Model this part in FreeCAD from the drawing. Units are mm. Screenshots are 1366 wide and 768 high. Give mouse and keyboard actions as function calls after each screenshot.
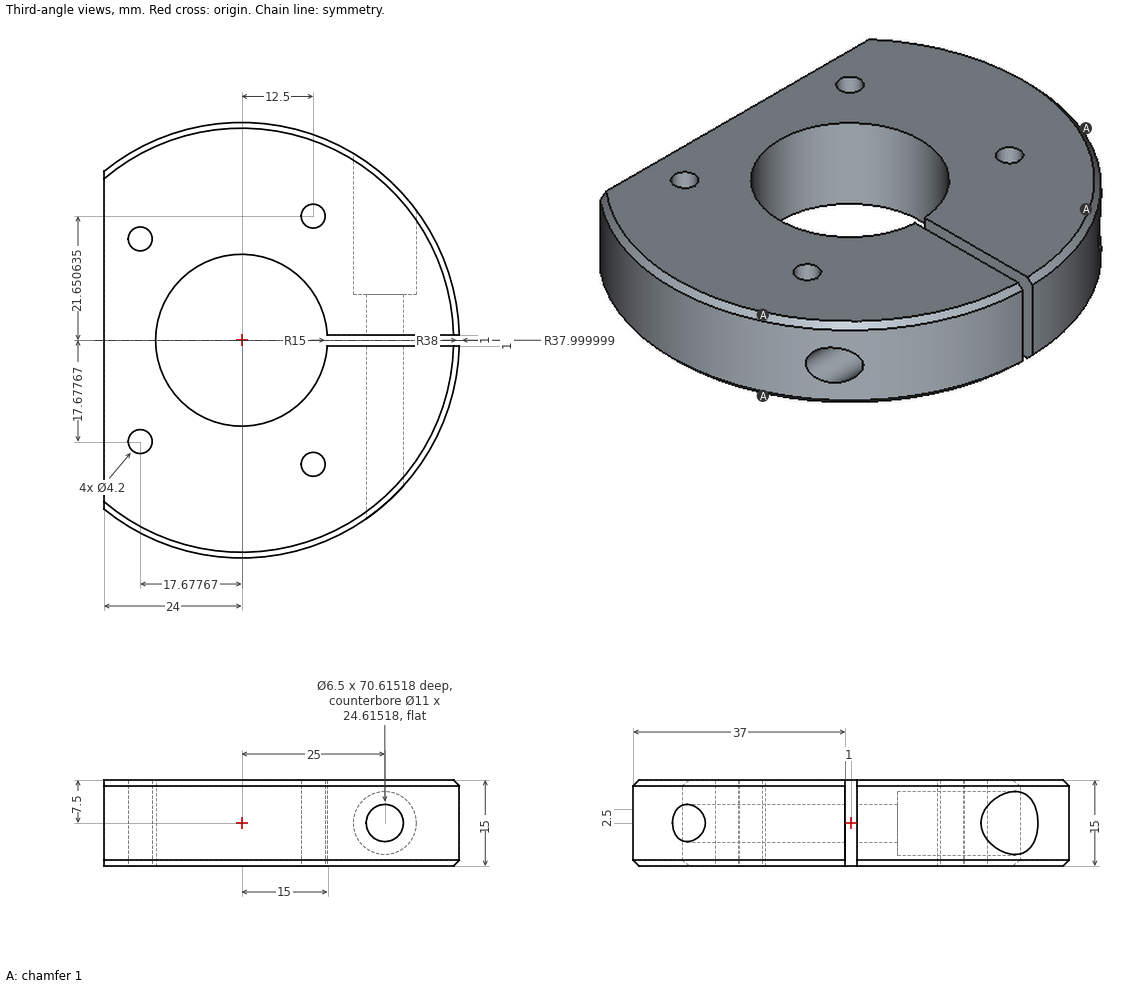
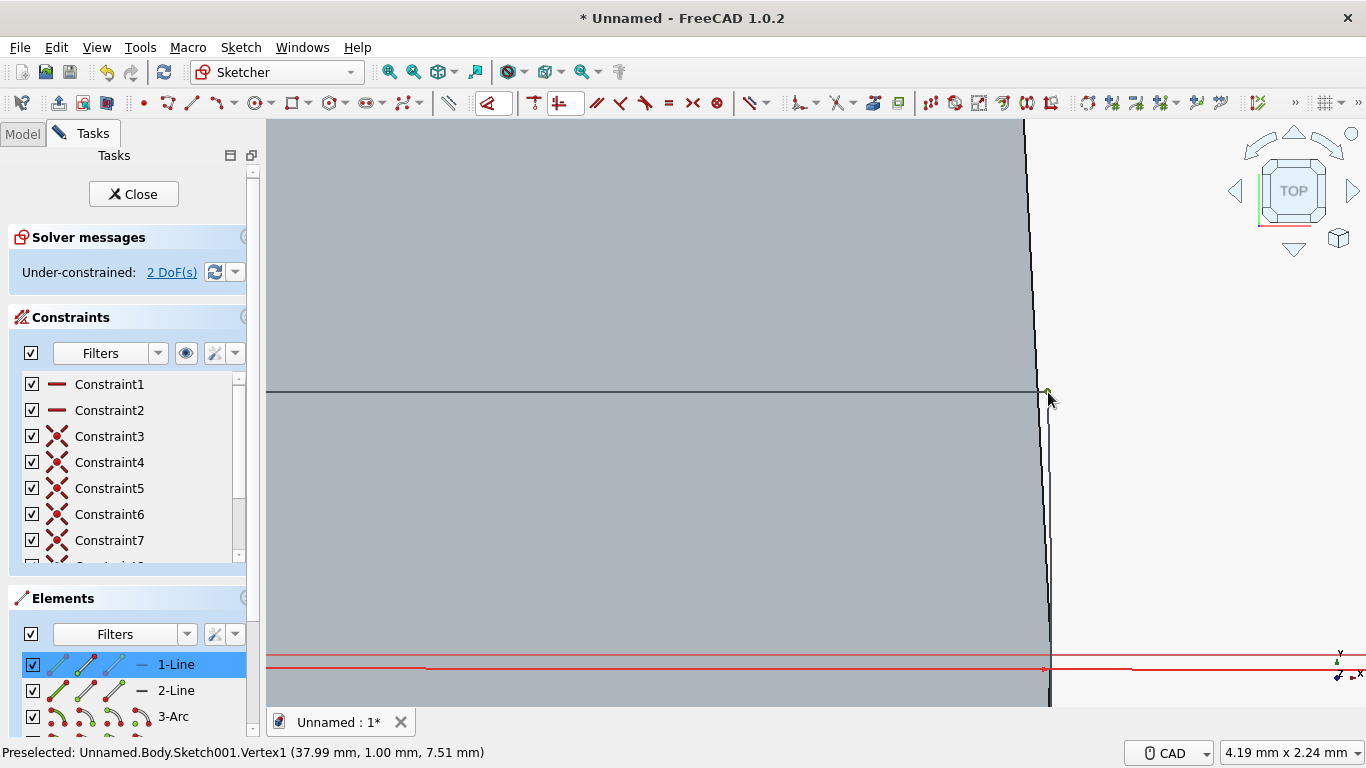
click(506, 104)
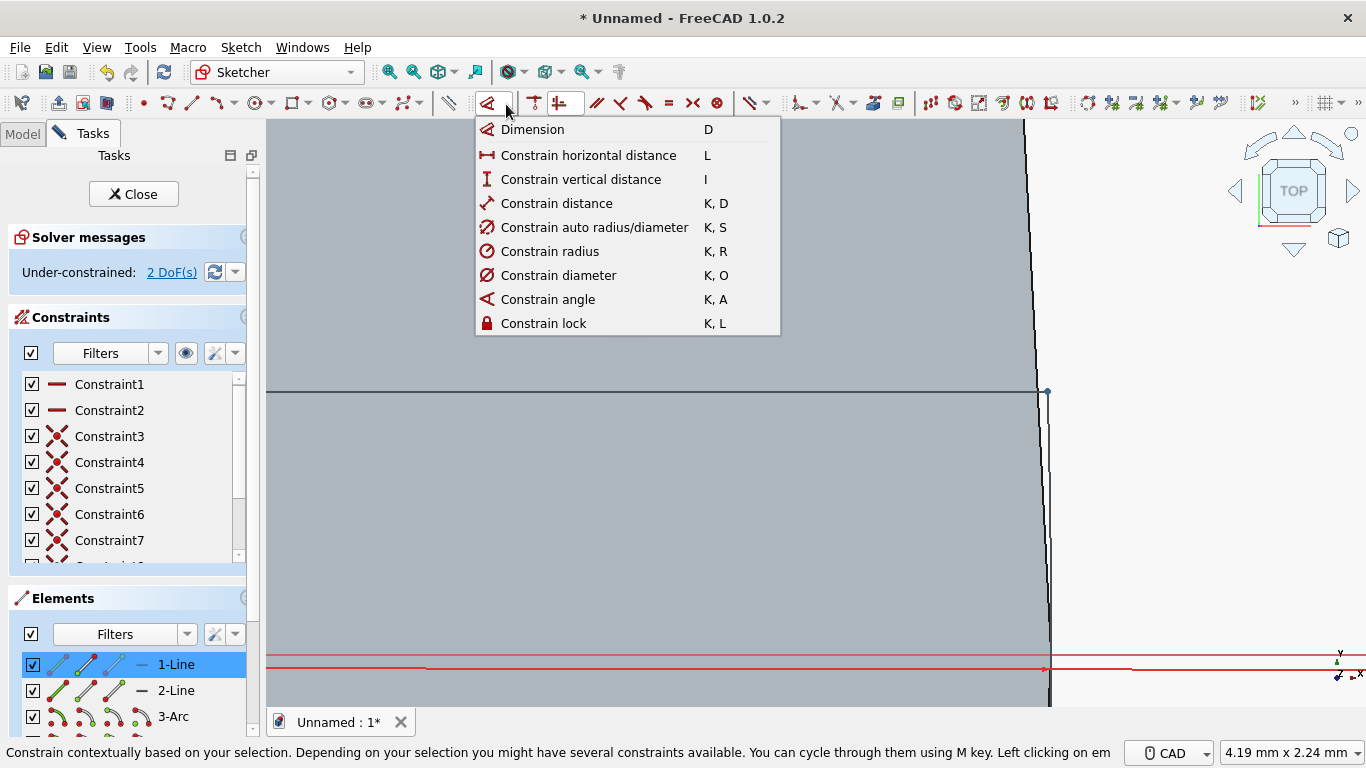
click(628, 179)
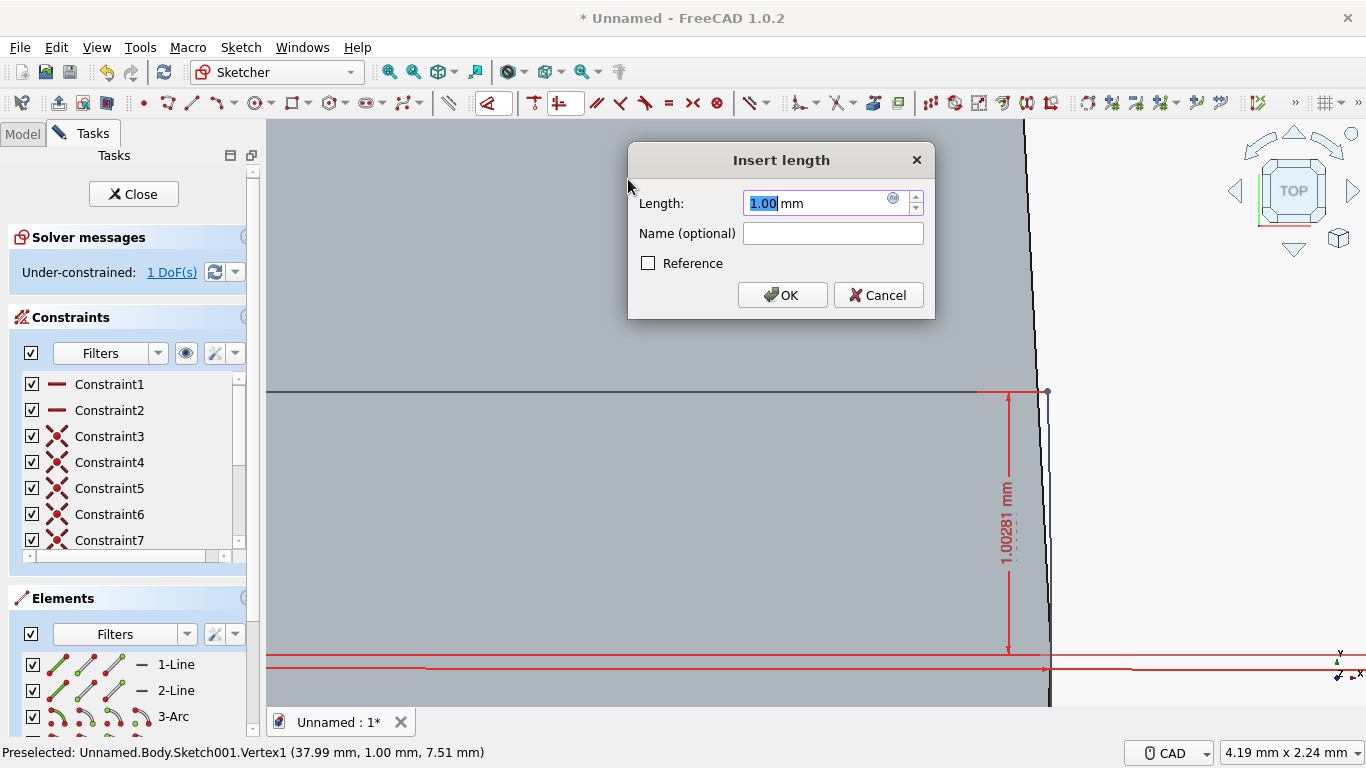
text(1)
key(Return)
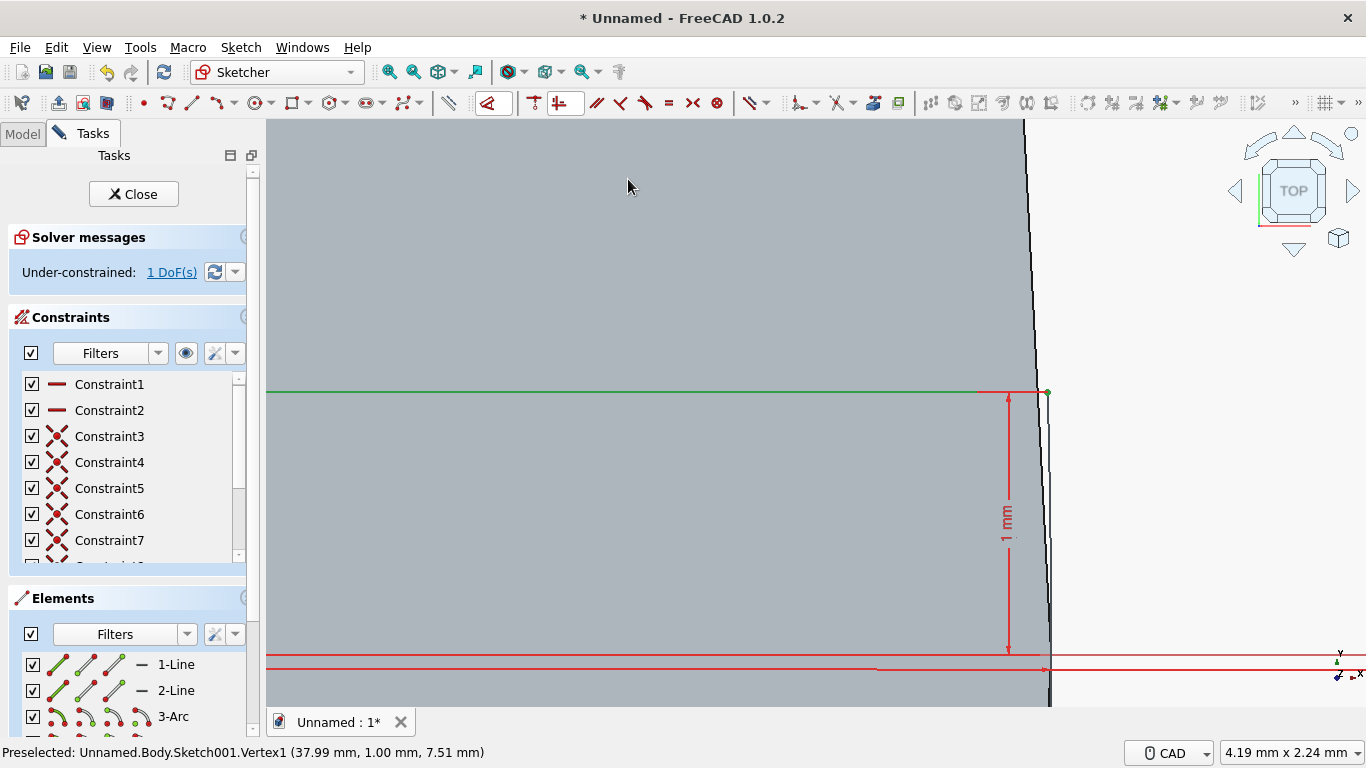
scroll(1051, 397, down, 14)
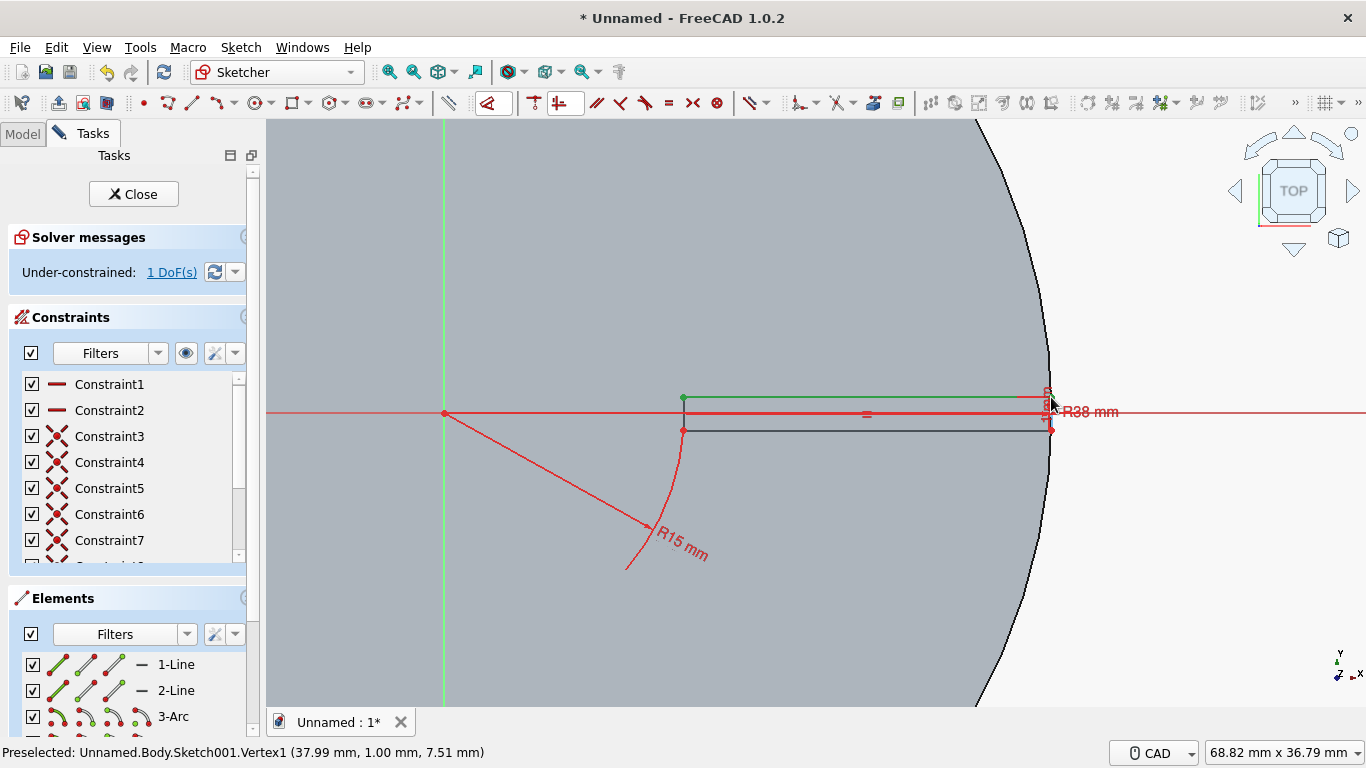
scroll(683, 431, up, 5)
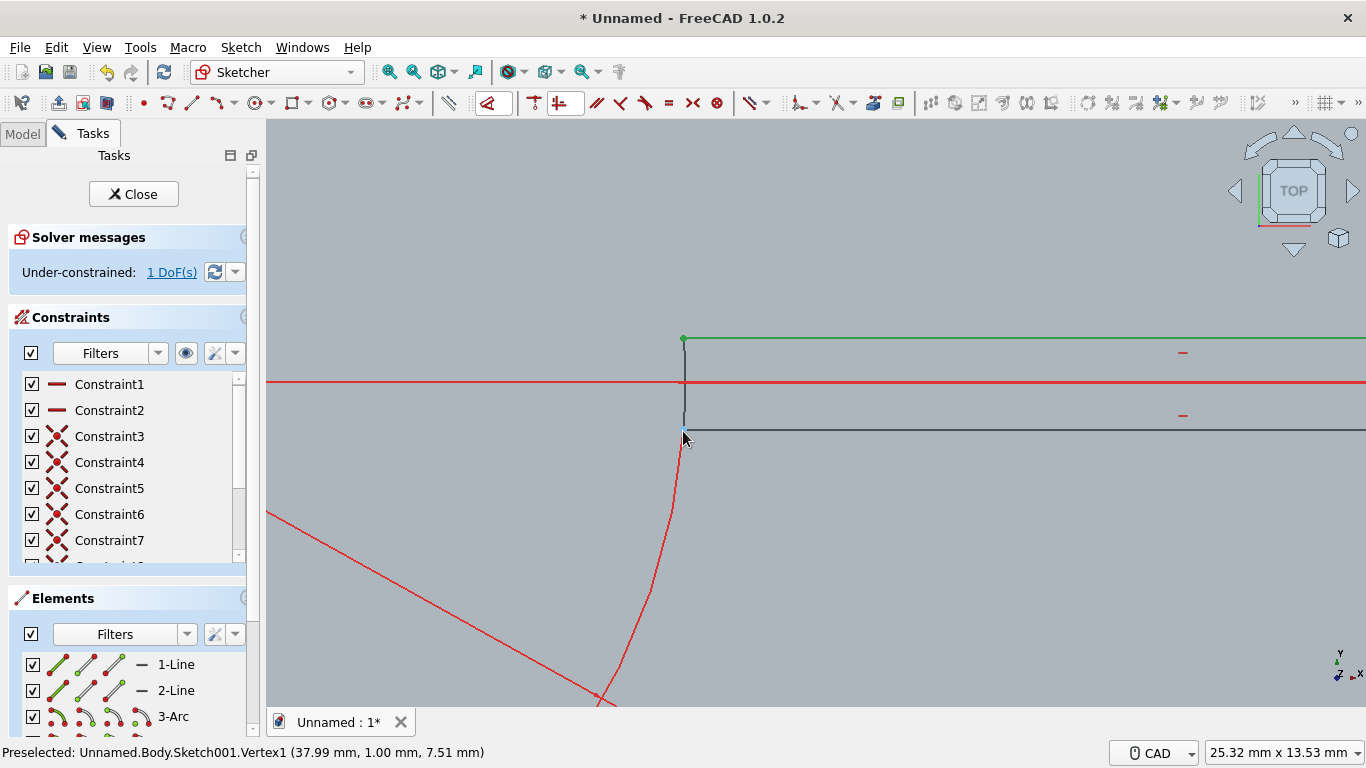
click(683, 430)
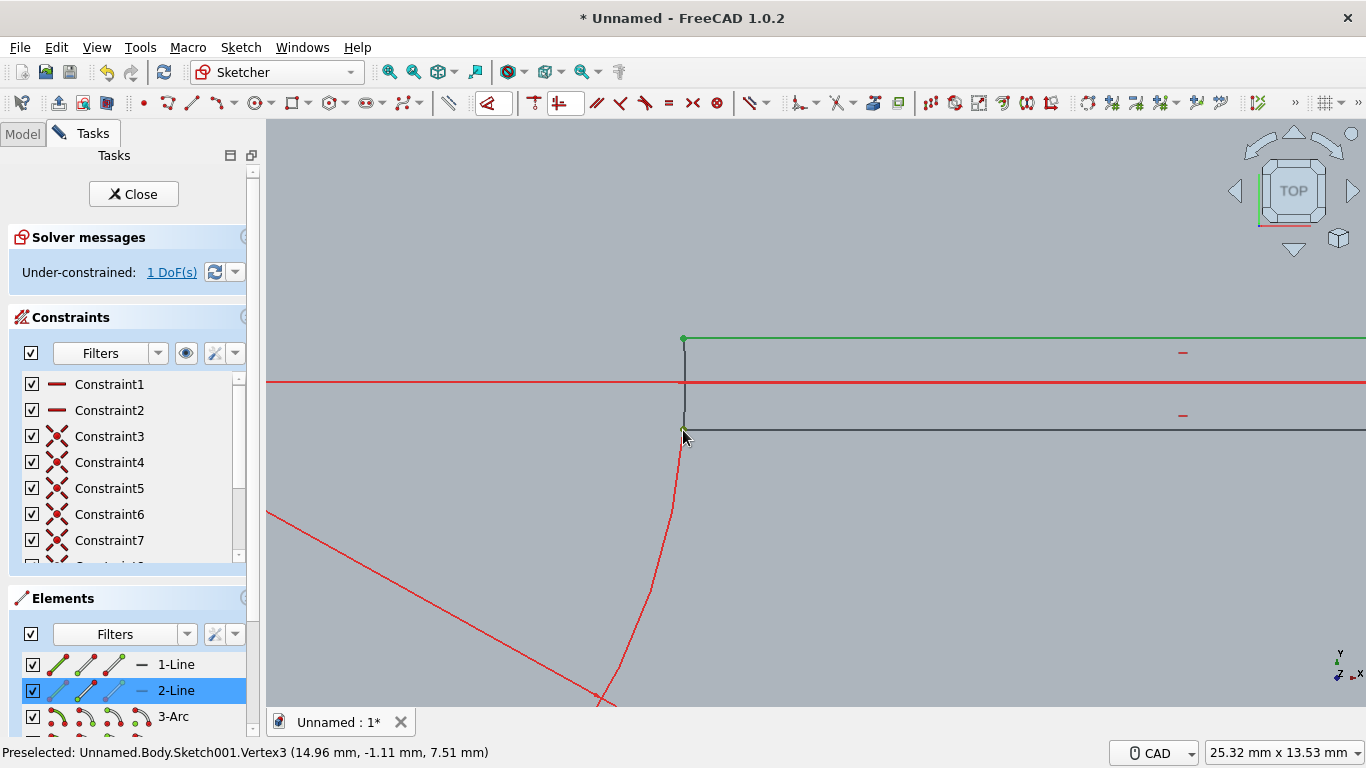
click(506, 104)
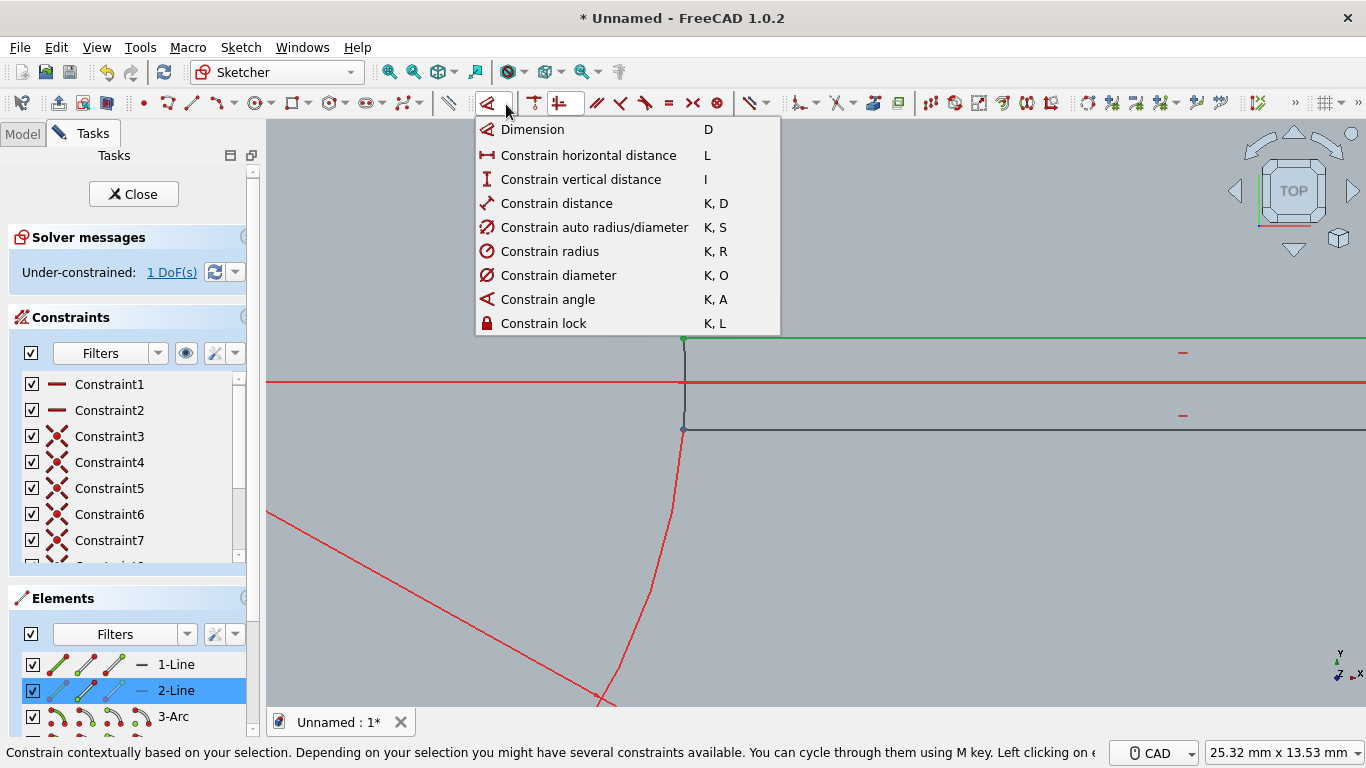
click(628, 179)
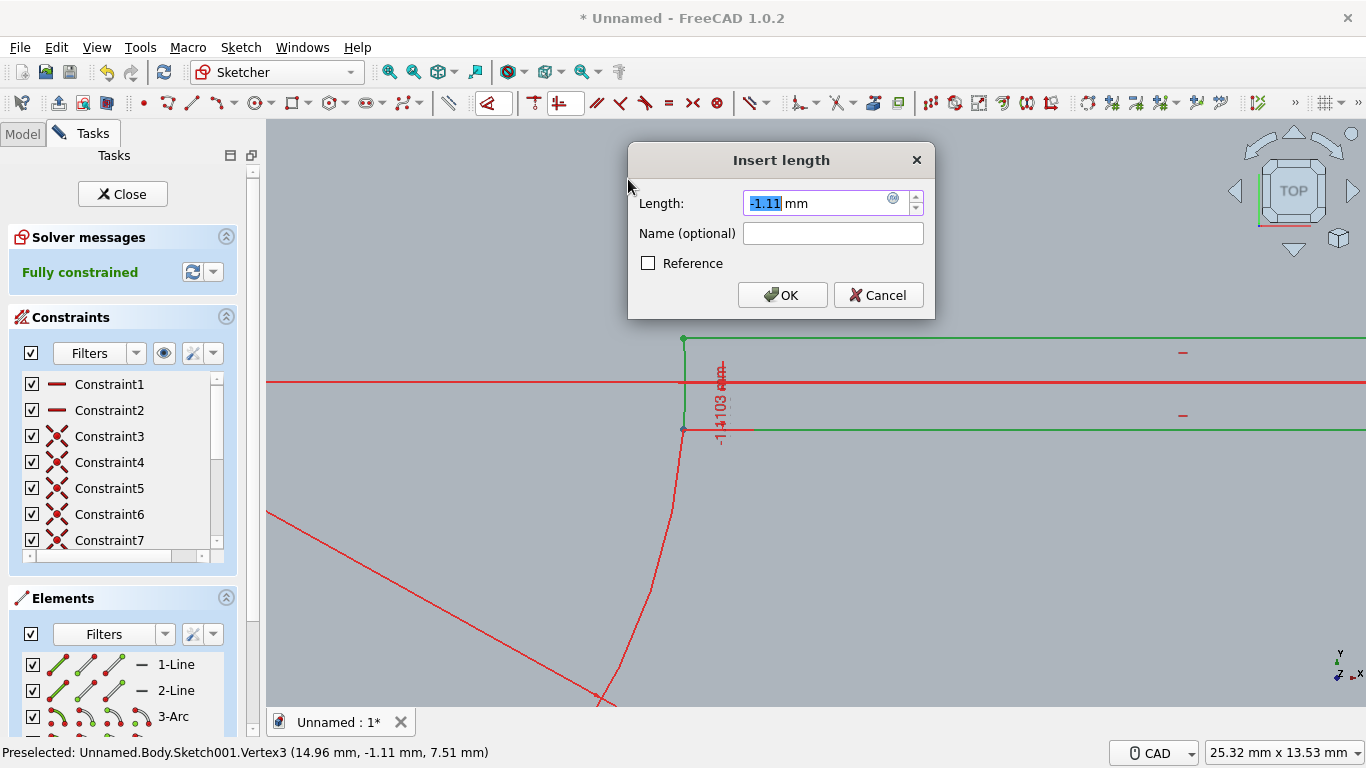
text(-1)
key(Return)